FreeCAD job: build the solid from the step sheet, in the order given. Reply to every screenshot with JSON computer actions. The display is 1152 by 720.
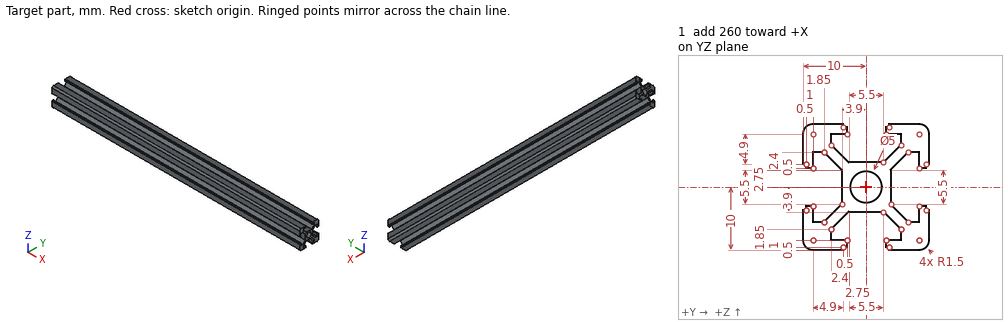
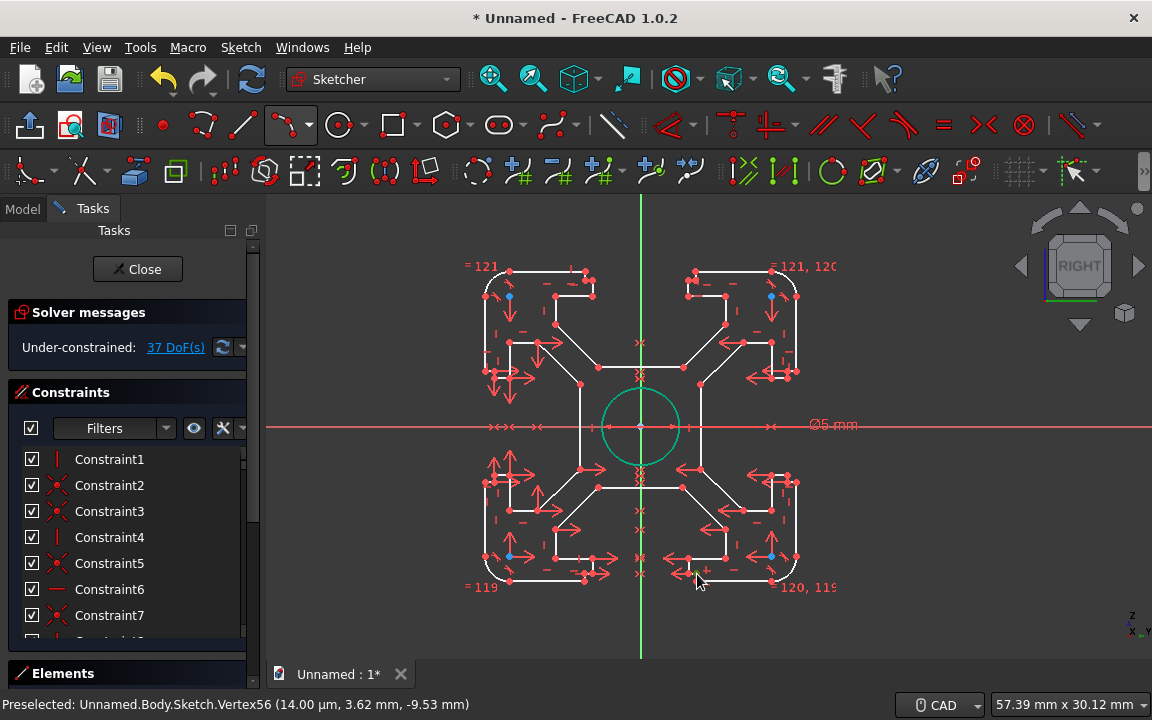
{"action": "scroll", "coordinate": [696, 280], "scroll_direction": "up", "scroll_amount": 3}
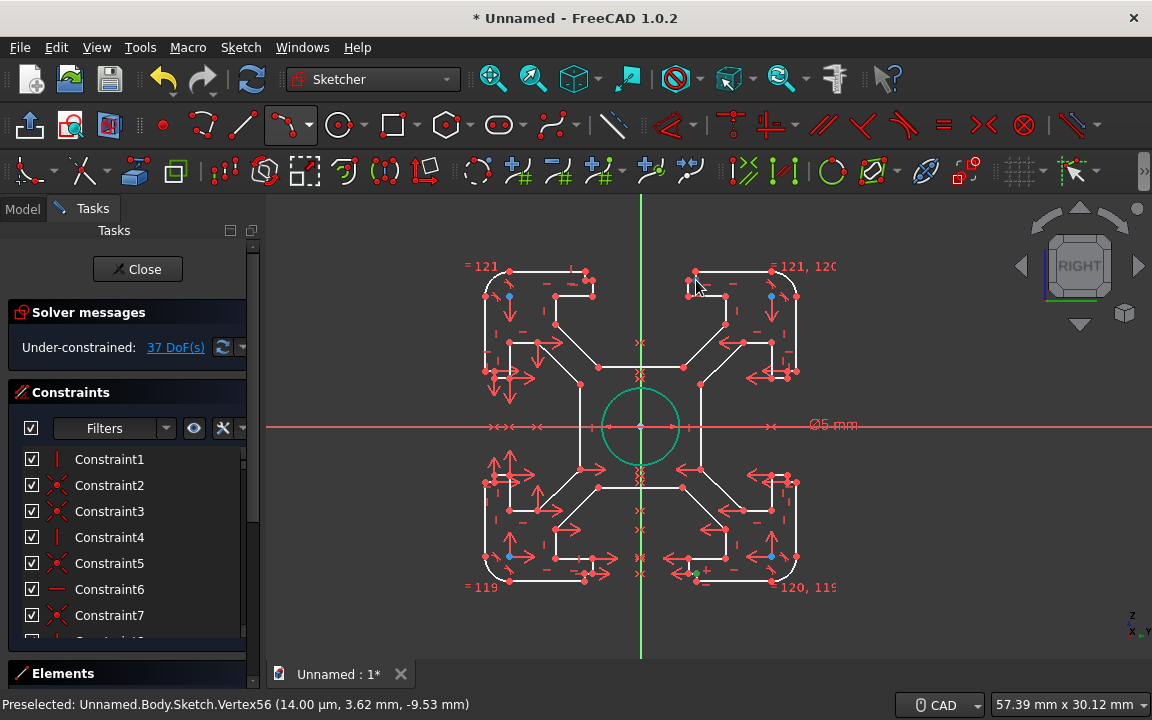
{"action": "left_click", "coordinate": [695, 280]}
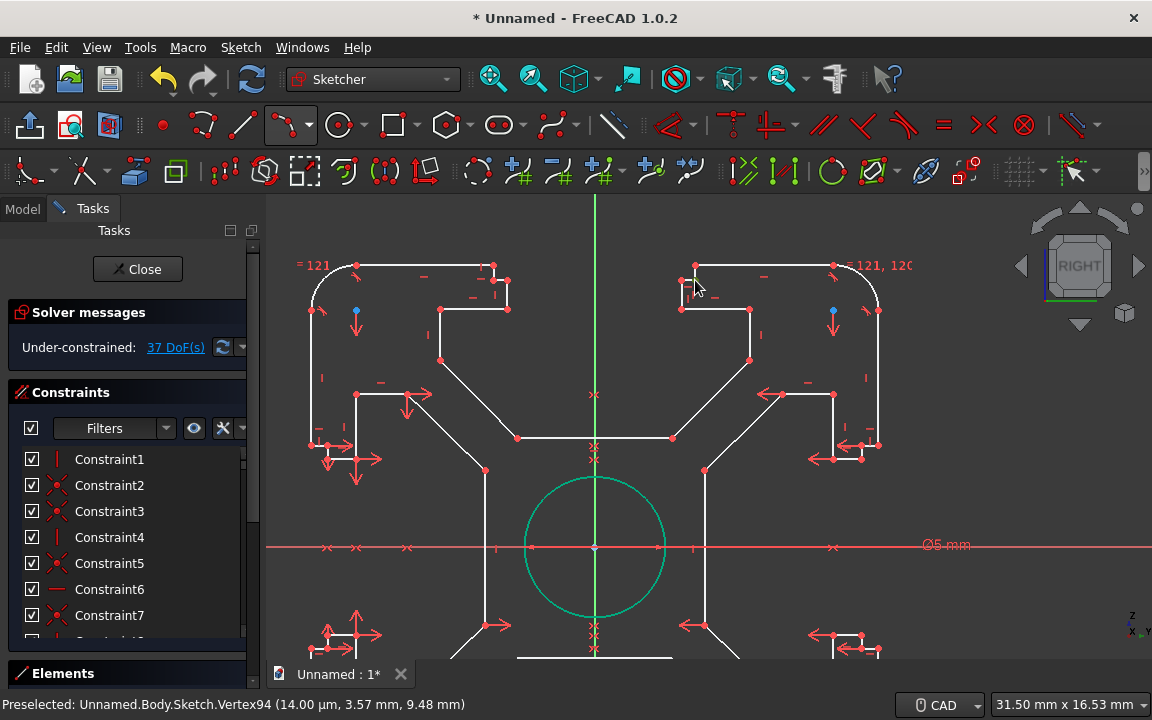
{"action": "left_click", "coordinate": [344, 547]}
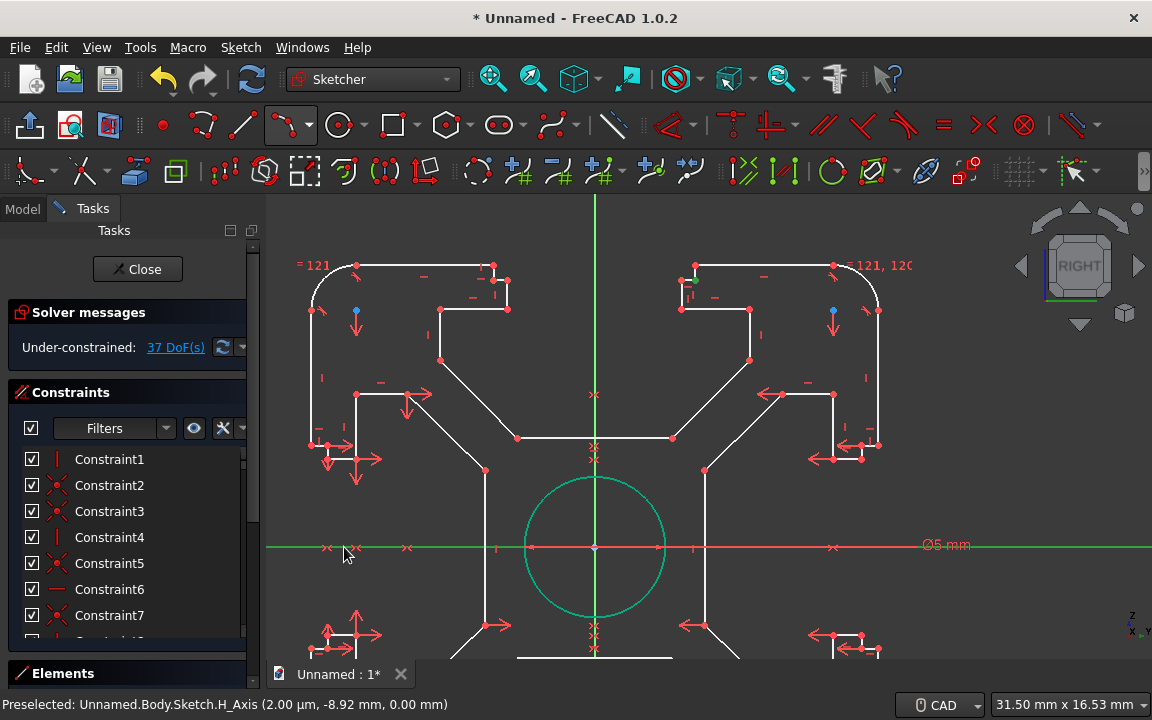
{"action": "key", "text": "s"}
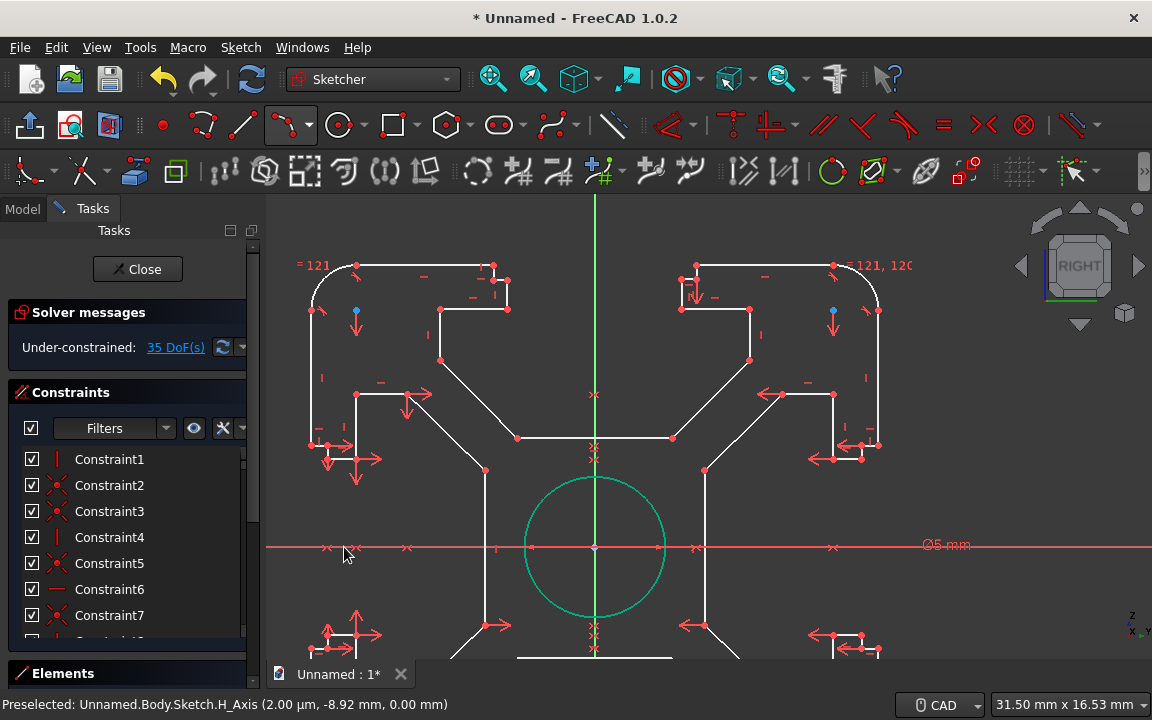
{"action": "scroll", "coordinate": [696, 280], "scroll_direction": "down", "scroll_amount": 3}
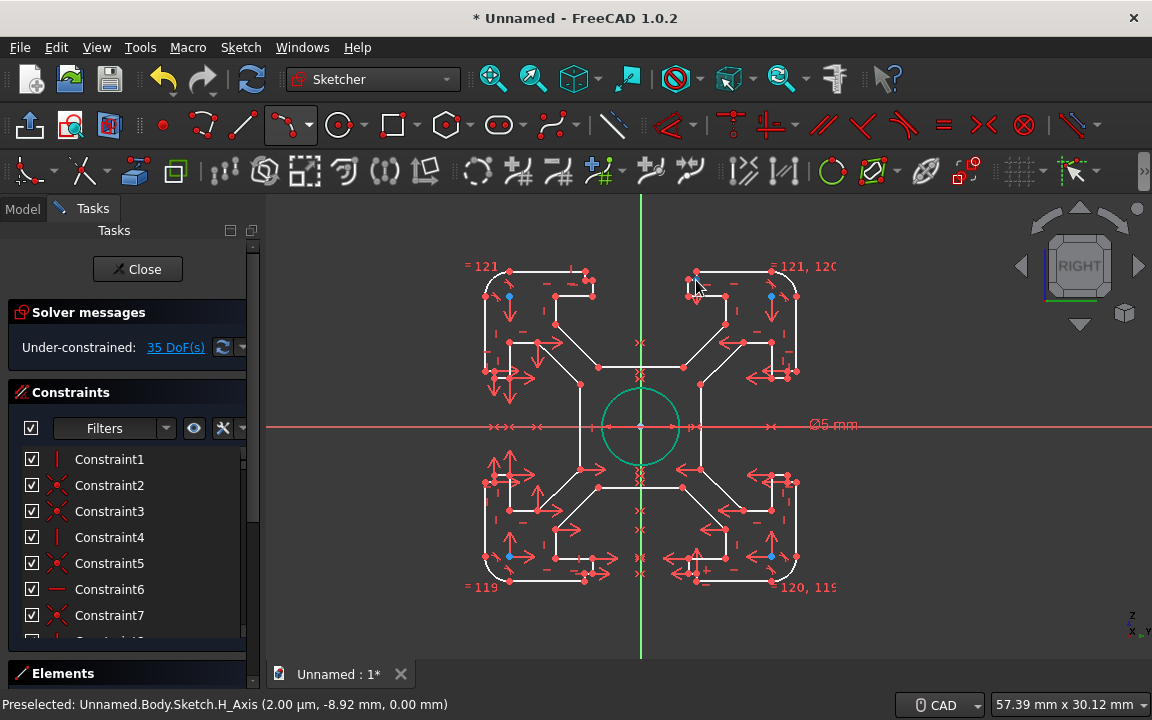
{"action": "left_click", "coordinate": [689, 559]}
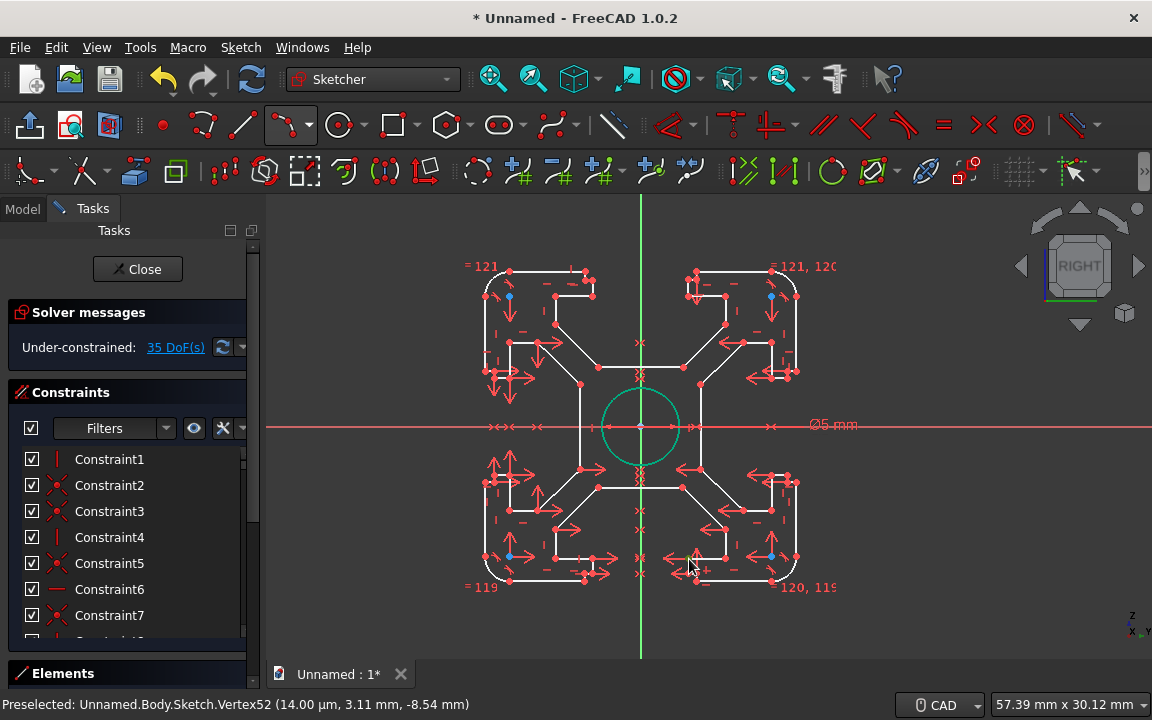
{"action": "left_click", "coordinate": [688, 296]}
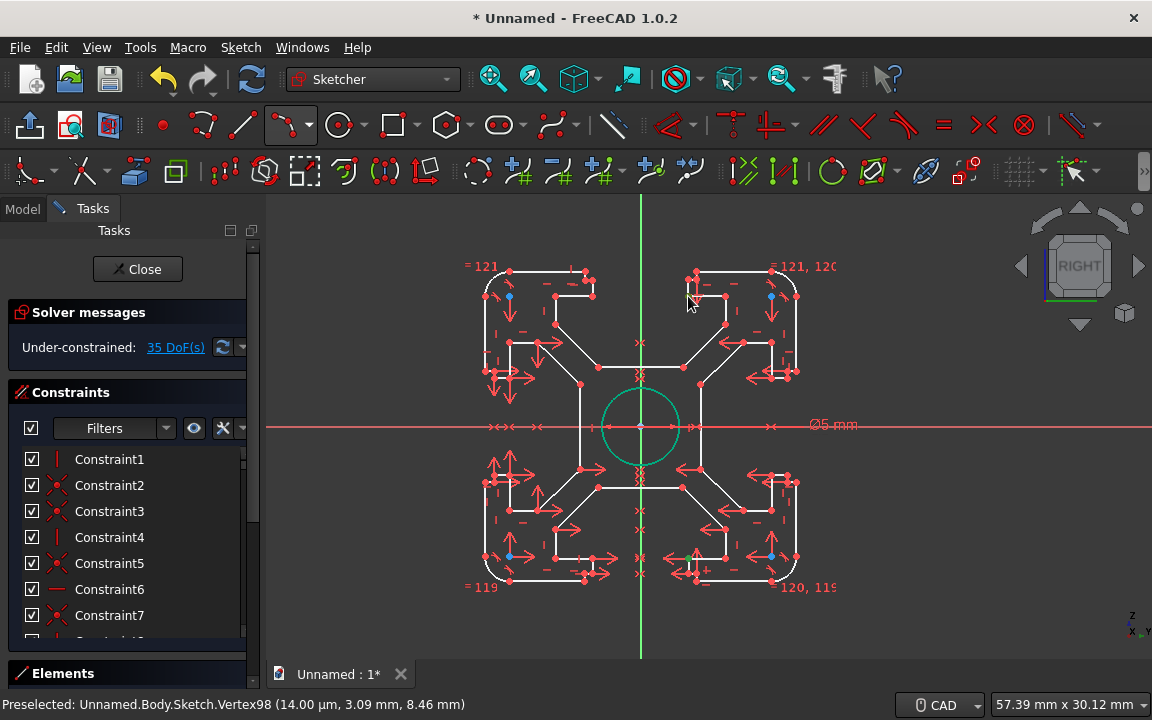
{"action": "left_click", "coordinate": [344, 427]}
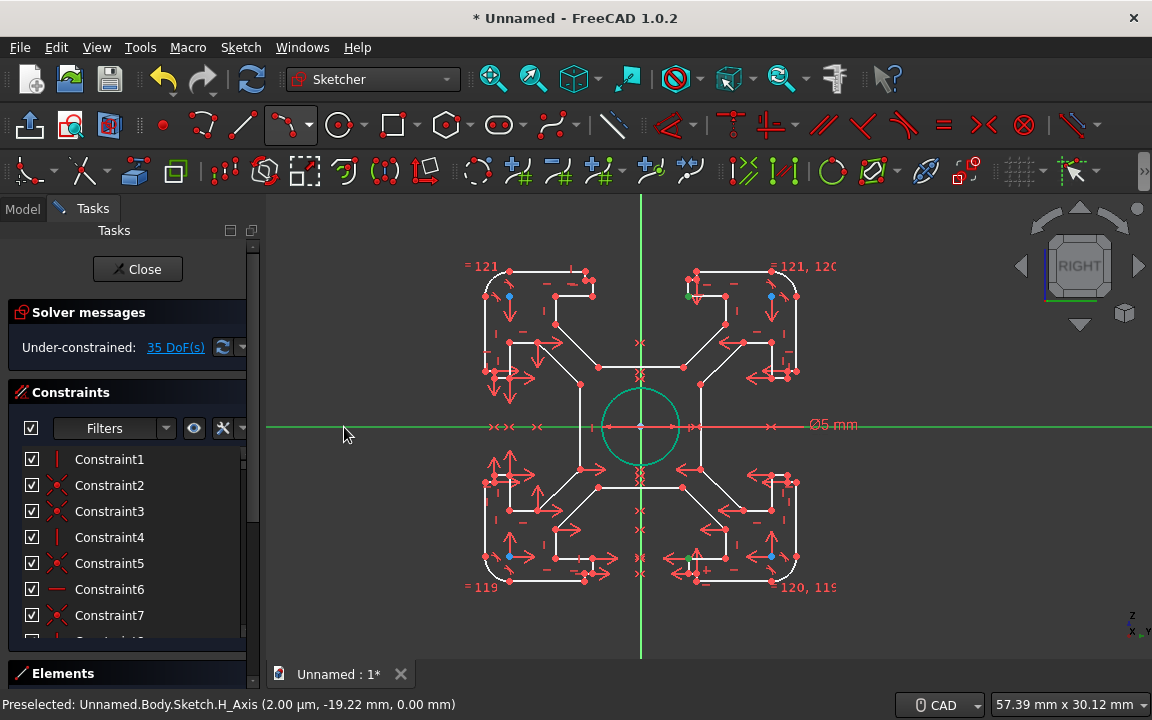
{"action": "left_click", "coordinate": [984, 126]}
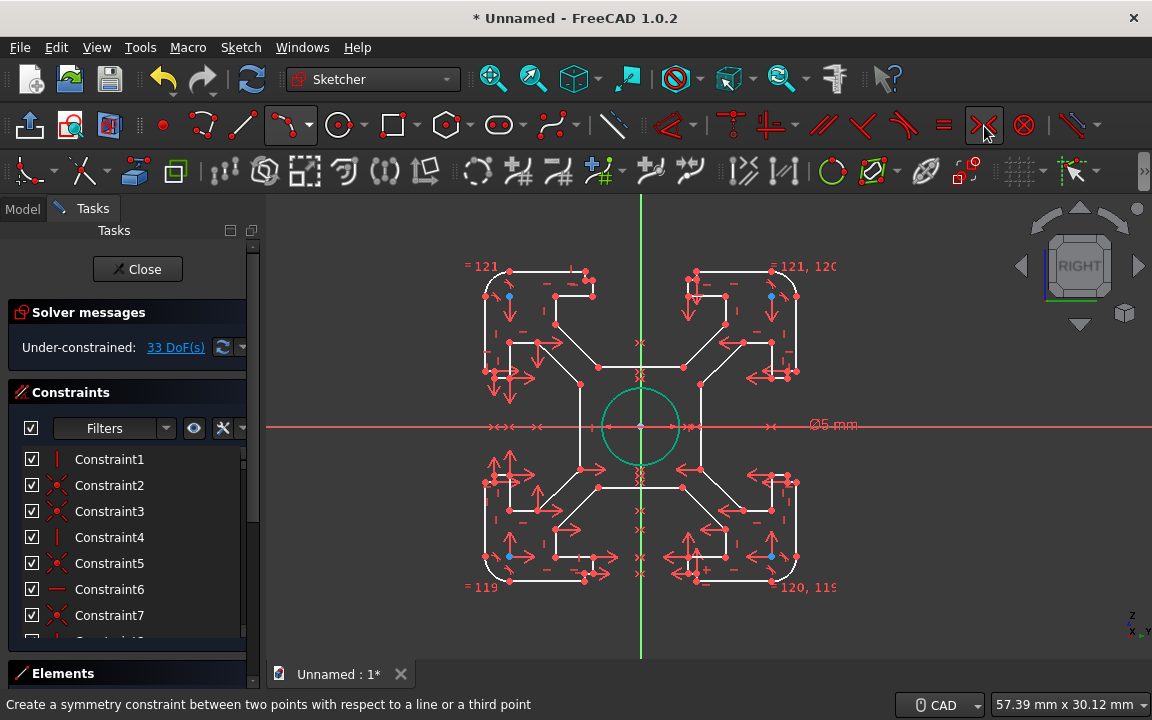
{"action": "left_click", "coordinate": [726, 530]}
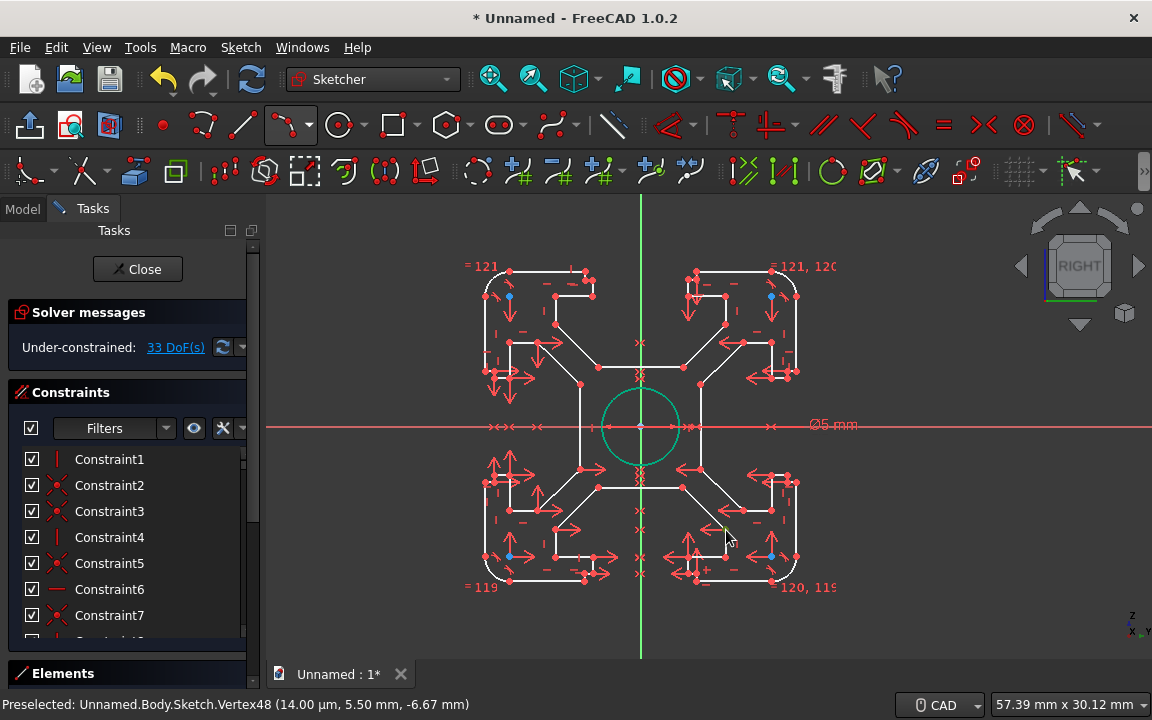
{"action": "left_click", "coordinate": [726, 324]}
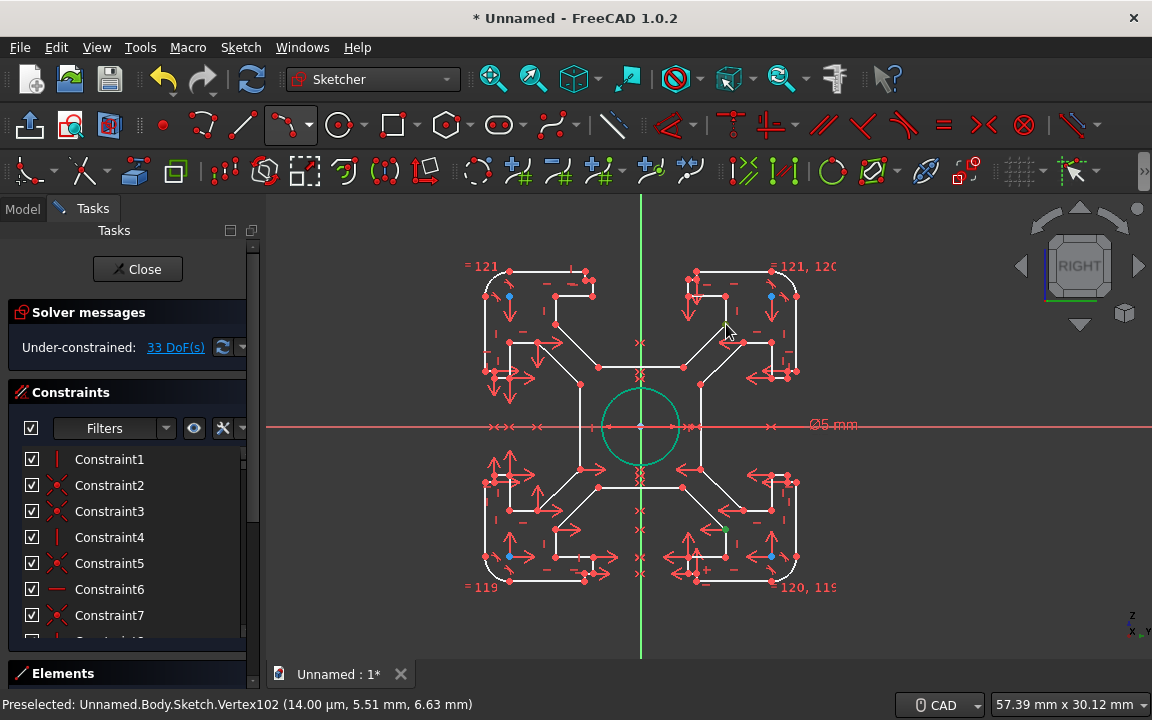
{"action": "left_click", "coordinate": [344, 427]}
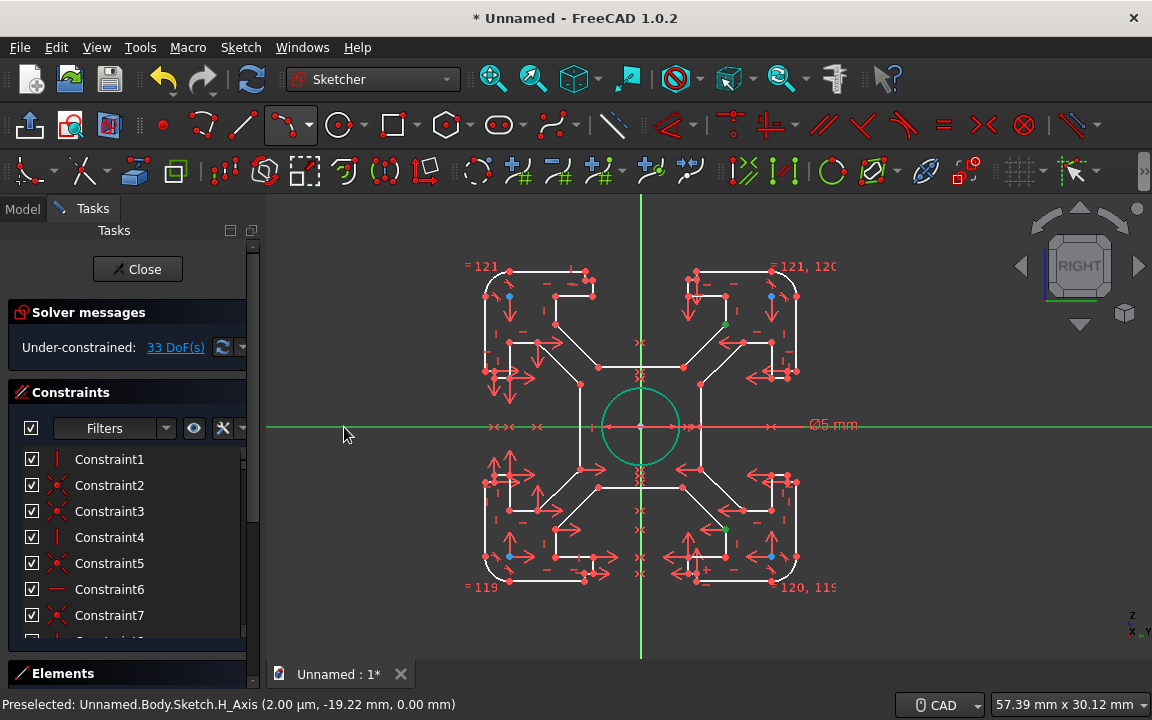
{"action": "key", "text": "s"}